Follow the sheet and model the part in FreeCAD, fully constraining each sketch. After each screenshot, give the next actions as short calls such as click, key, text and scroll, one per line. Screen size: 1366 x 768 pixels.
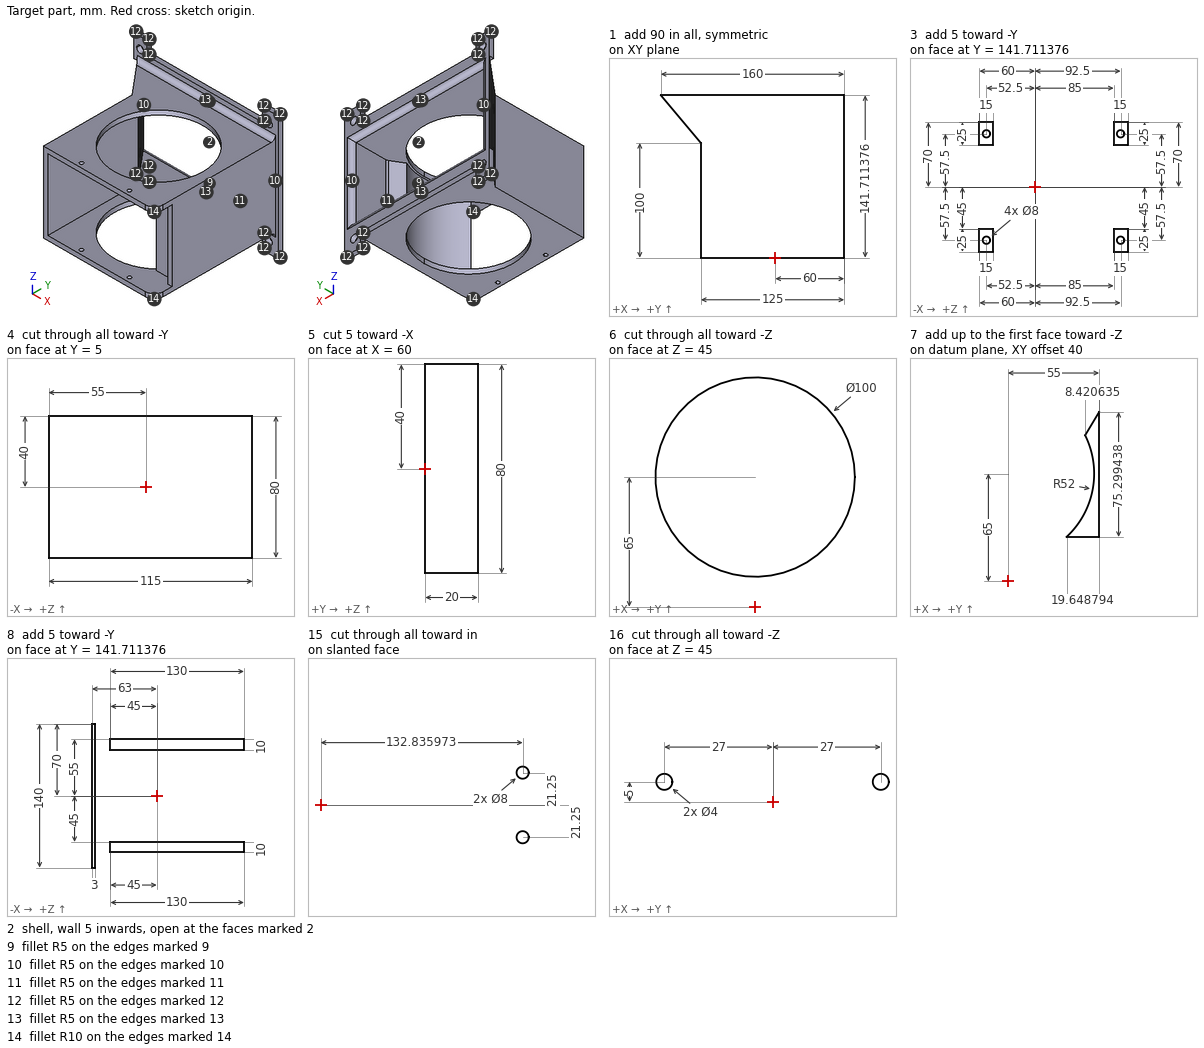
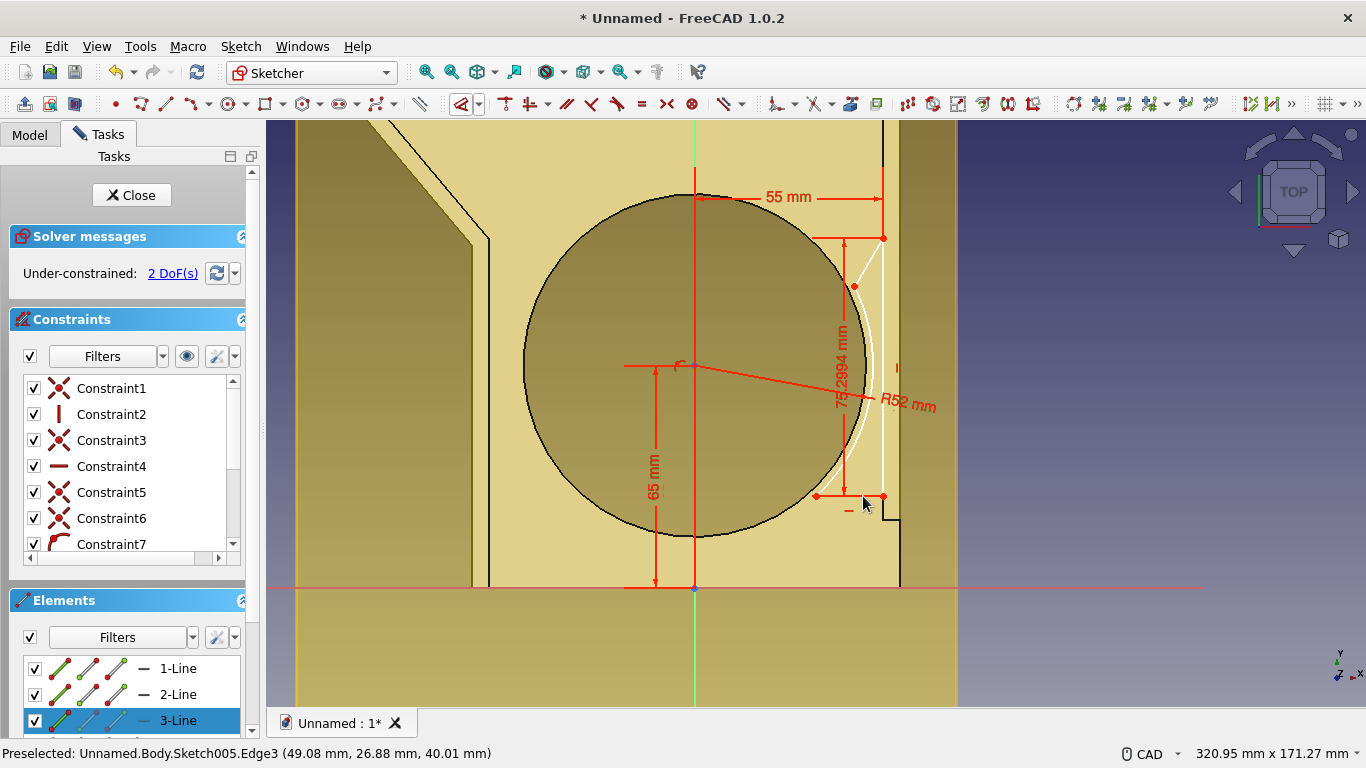
click(478, 104)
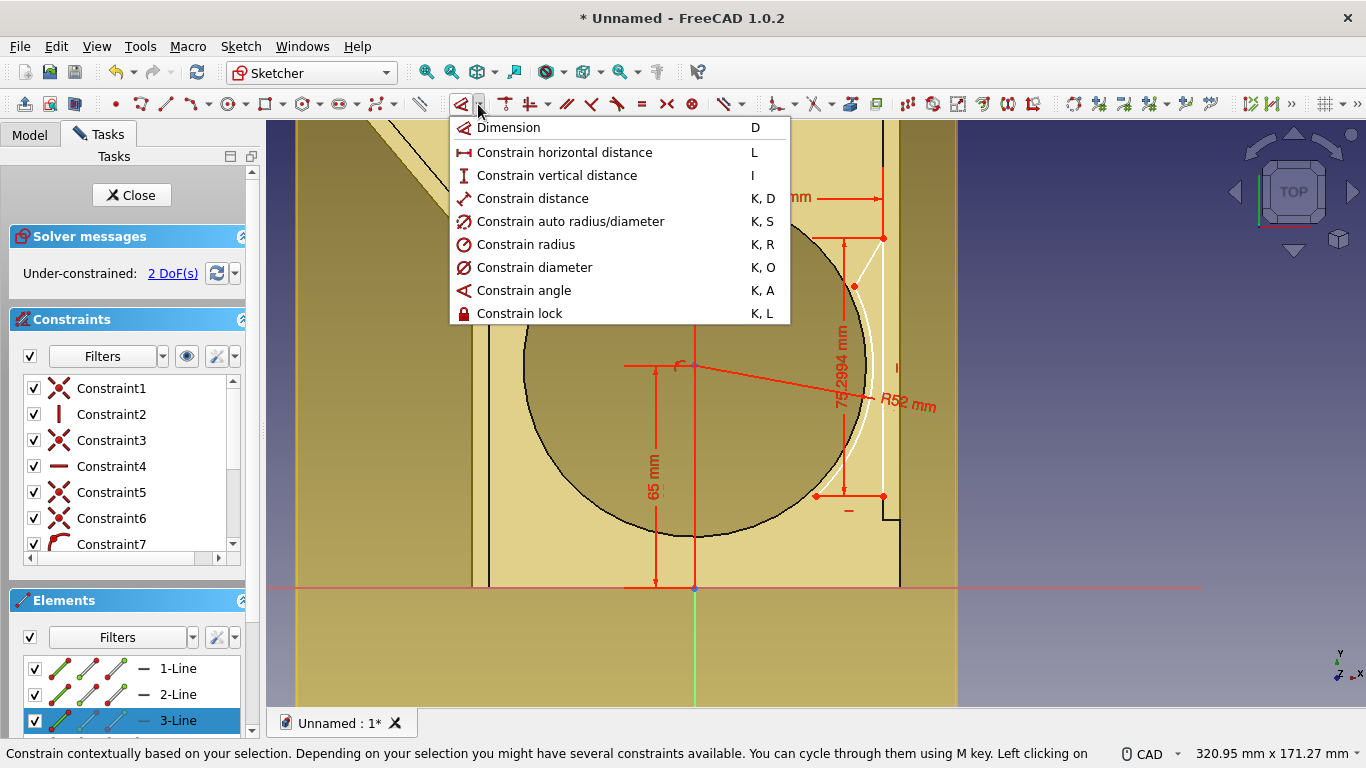
click(620, 152)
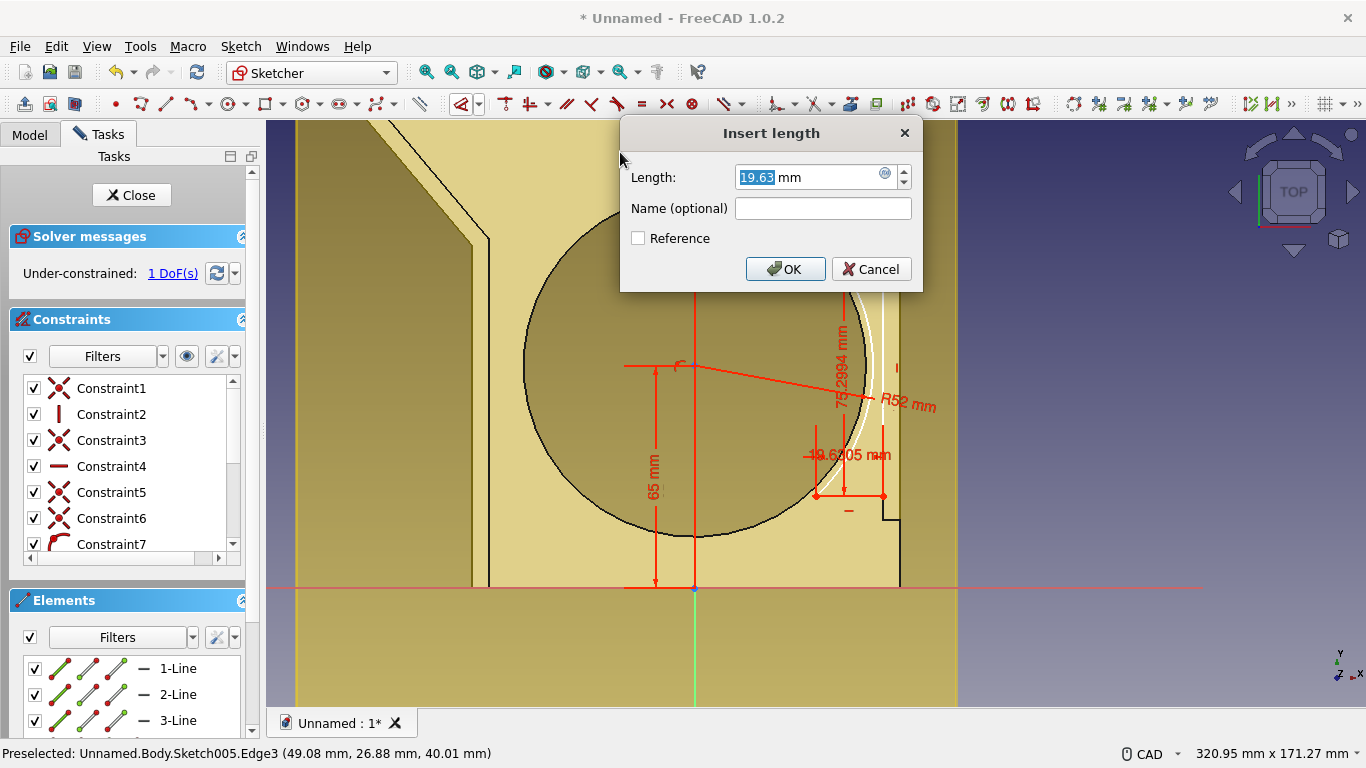
text(19.648794)
key(Return)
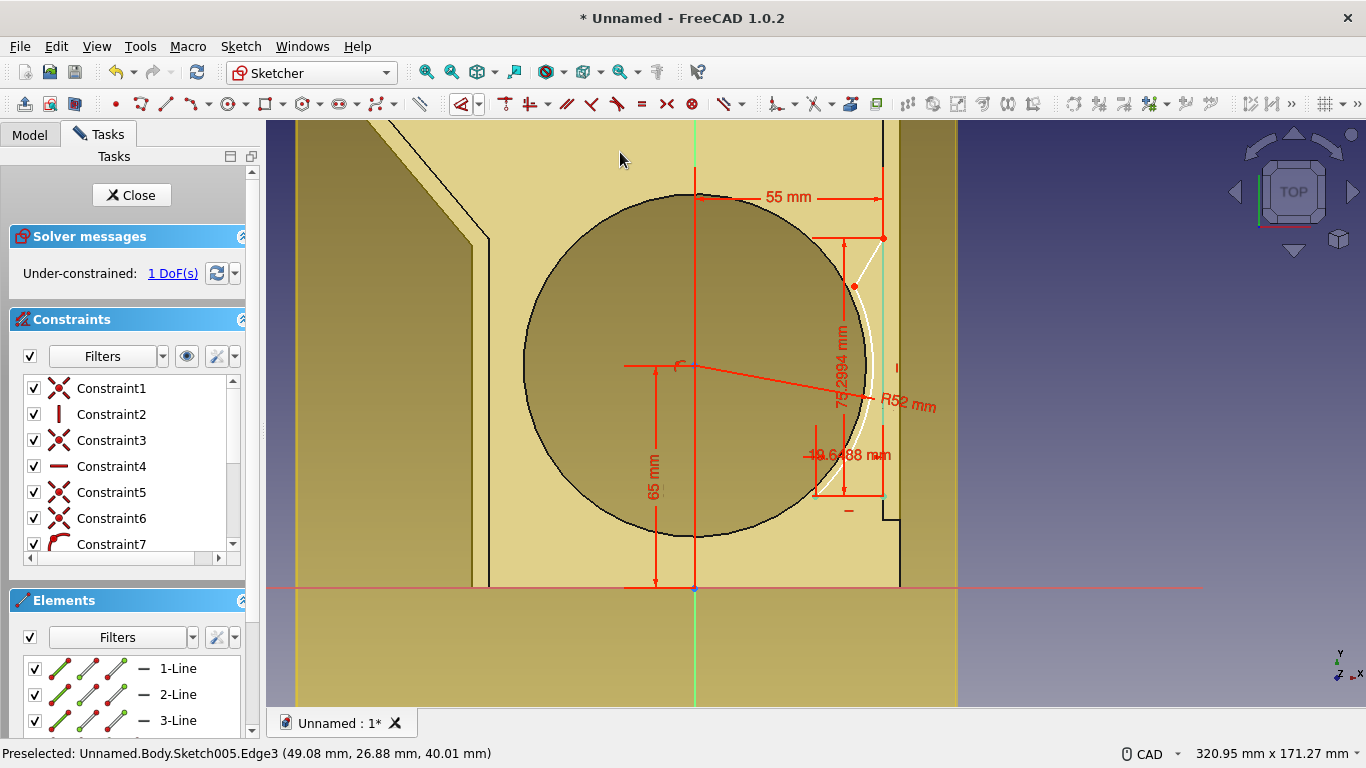
scroll(863, 272, up, 2)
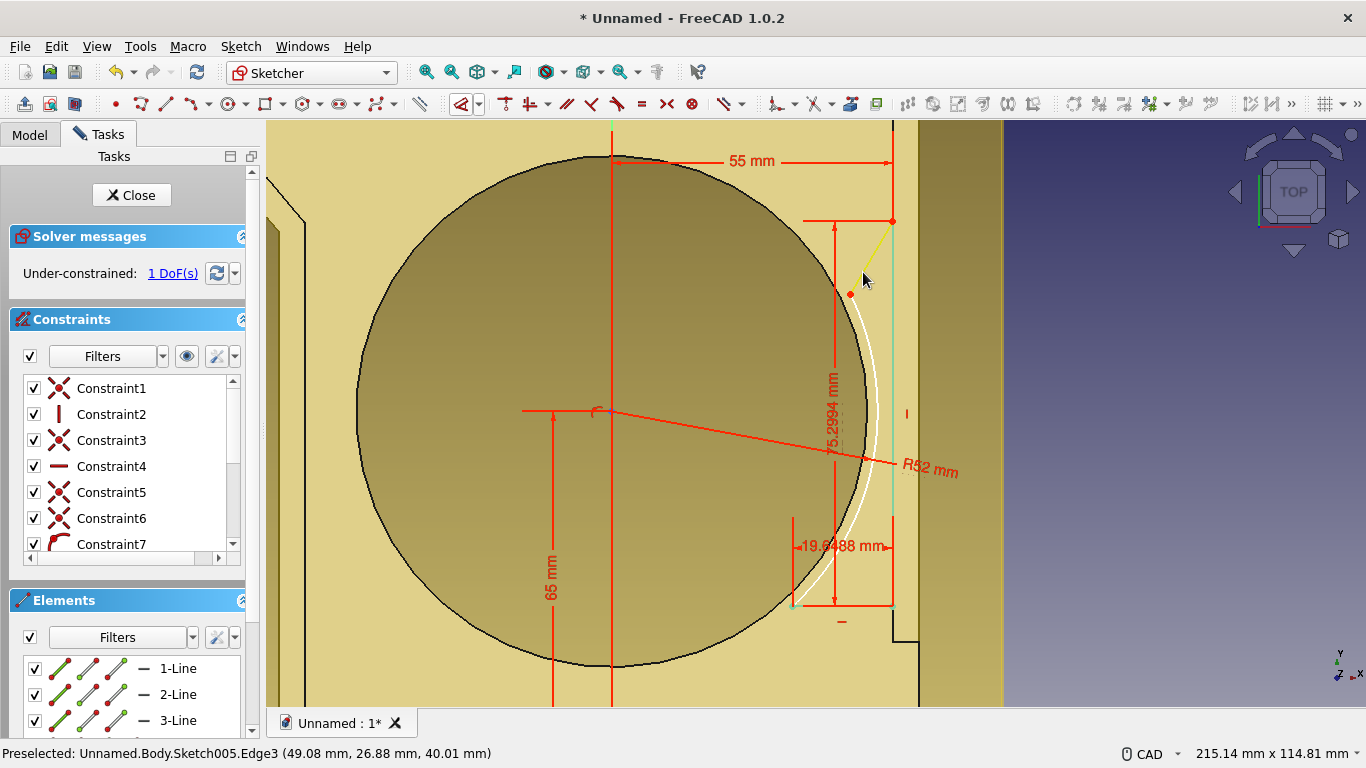
click(863, 272)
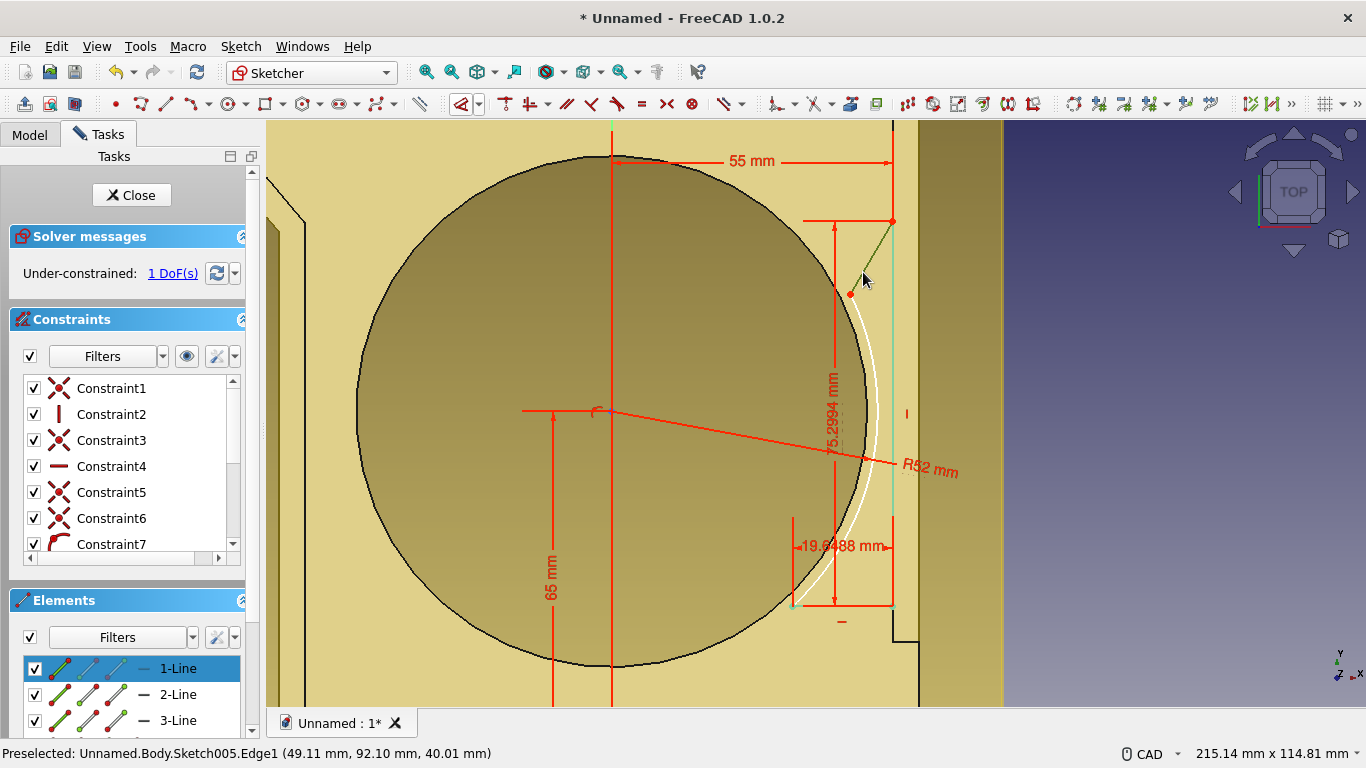
key(l)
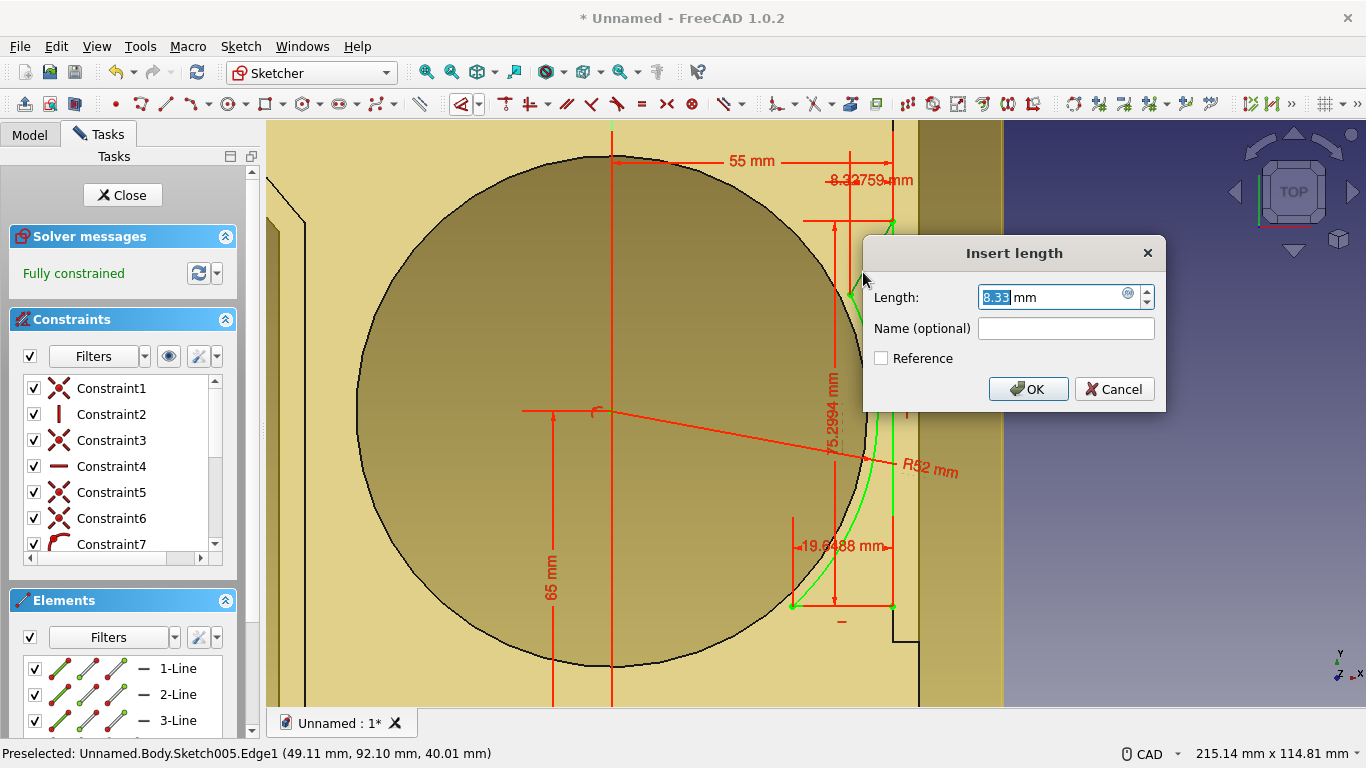
text(8.420635)
key(Return)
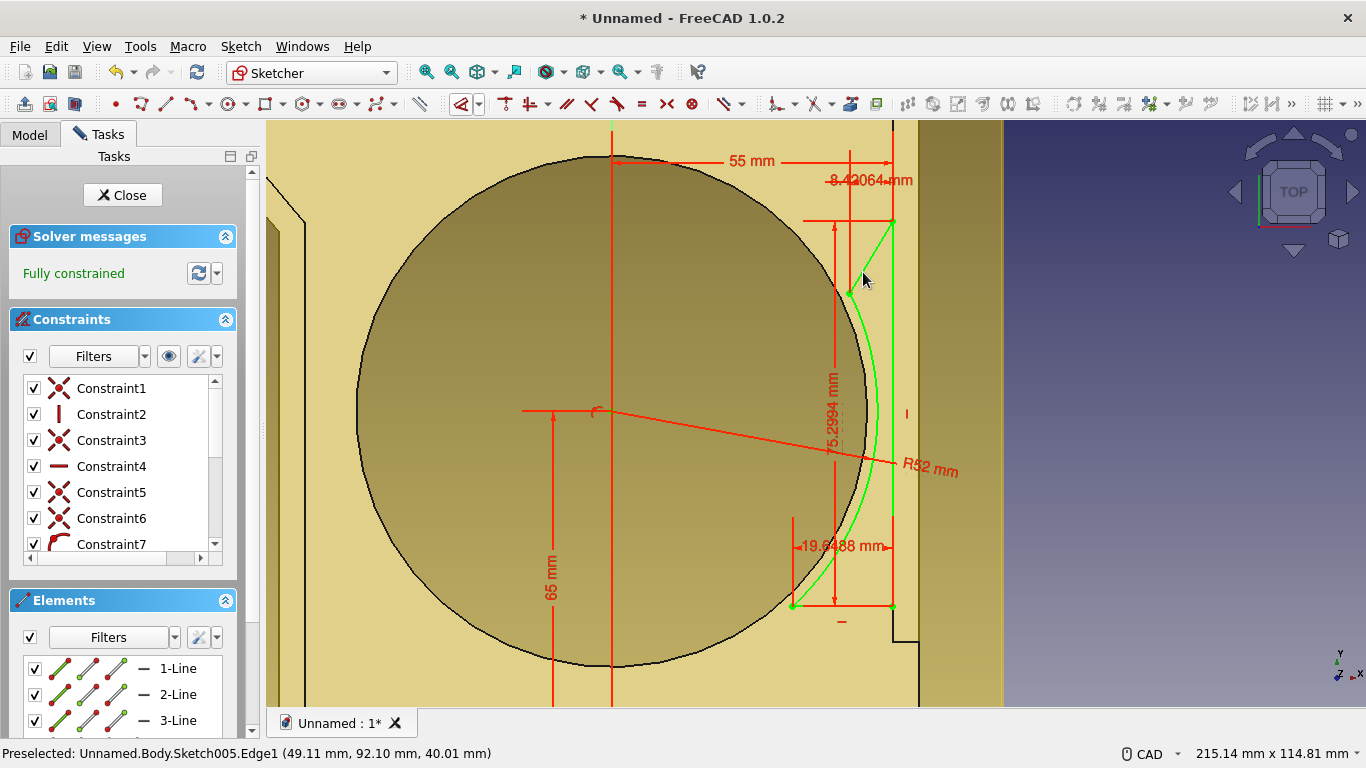
click(123, 195)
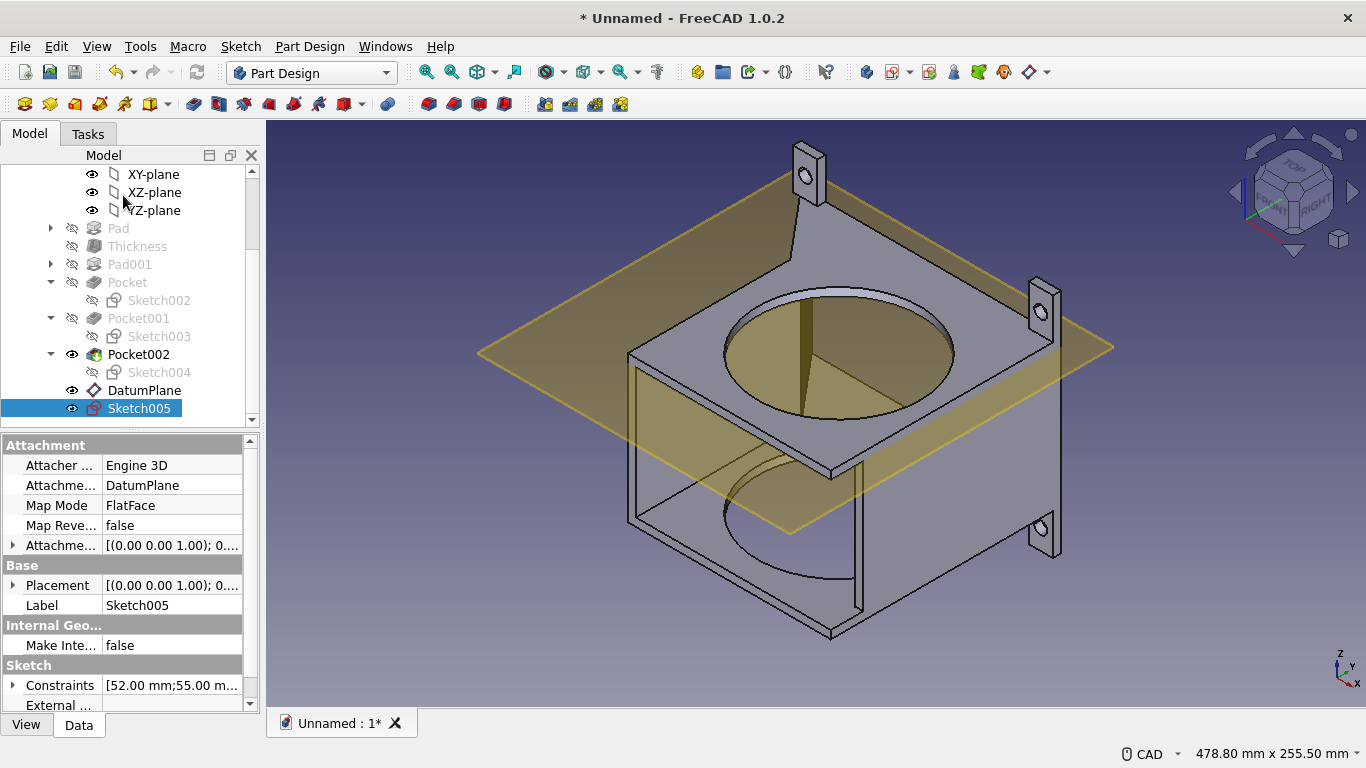
click(25, 104)